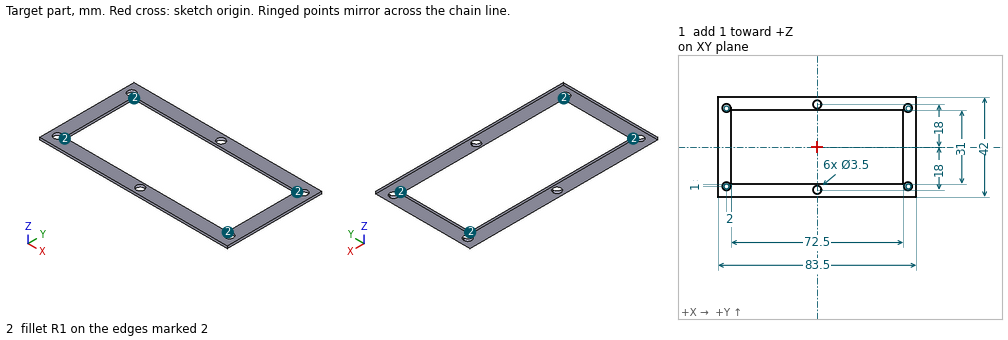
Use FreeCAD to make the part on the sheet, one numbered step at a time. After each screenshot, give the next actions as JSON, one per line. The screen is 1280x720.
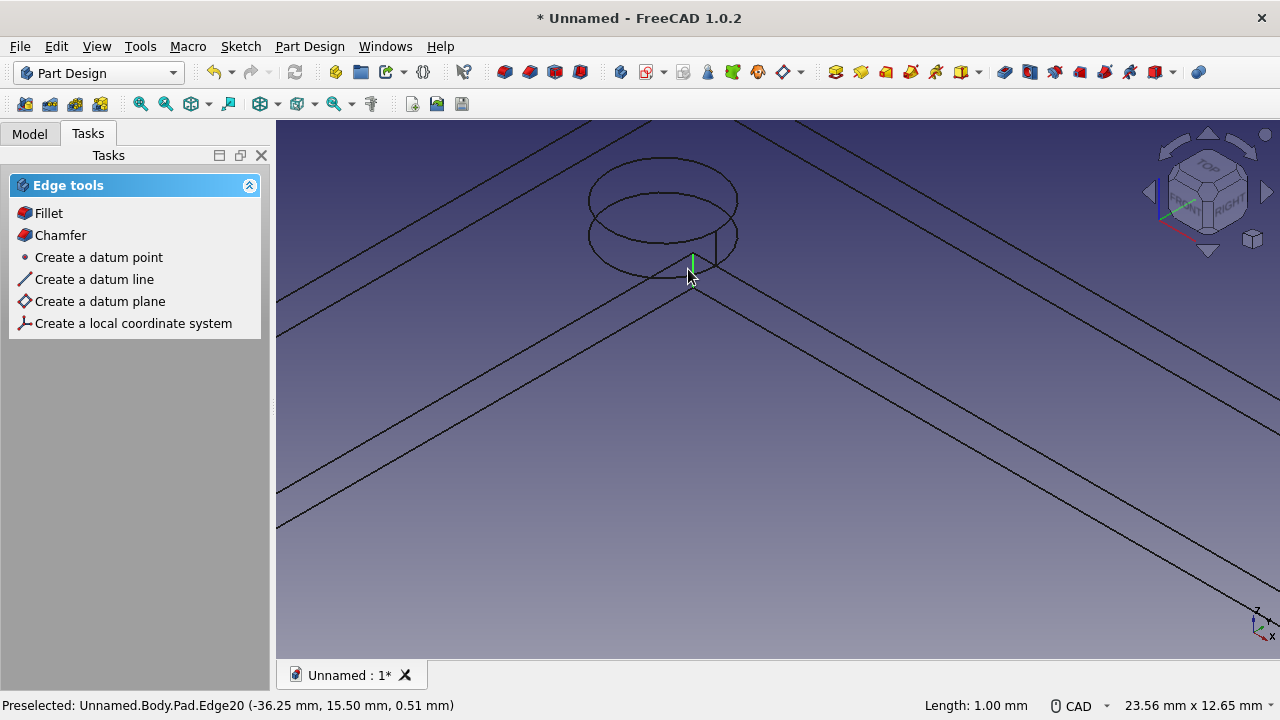
{"action": "key", "text": "v f"}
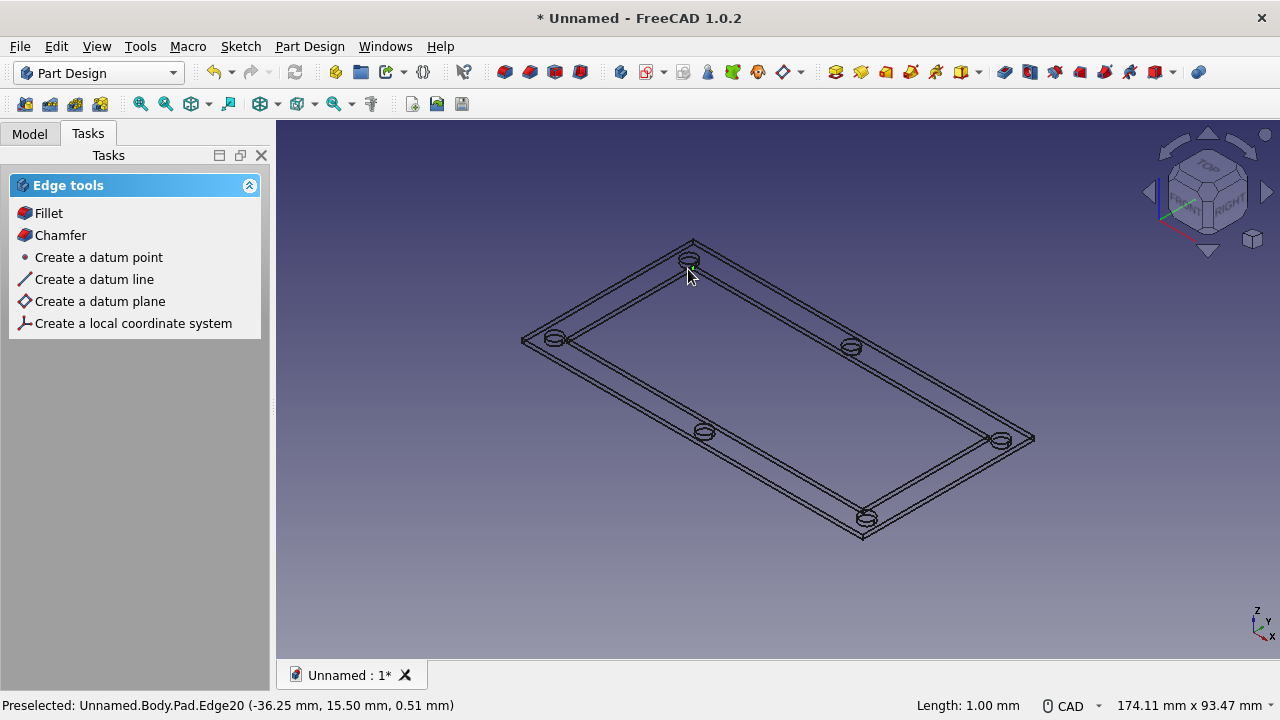
{"action": "key", "text": "2"}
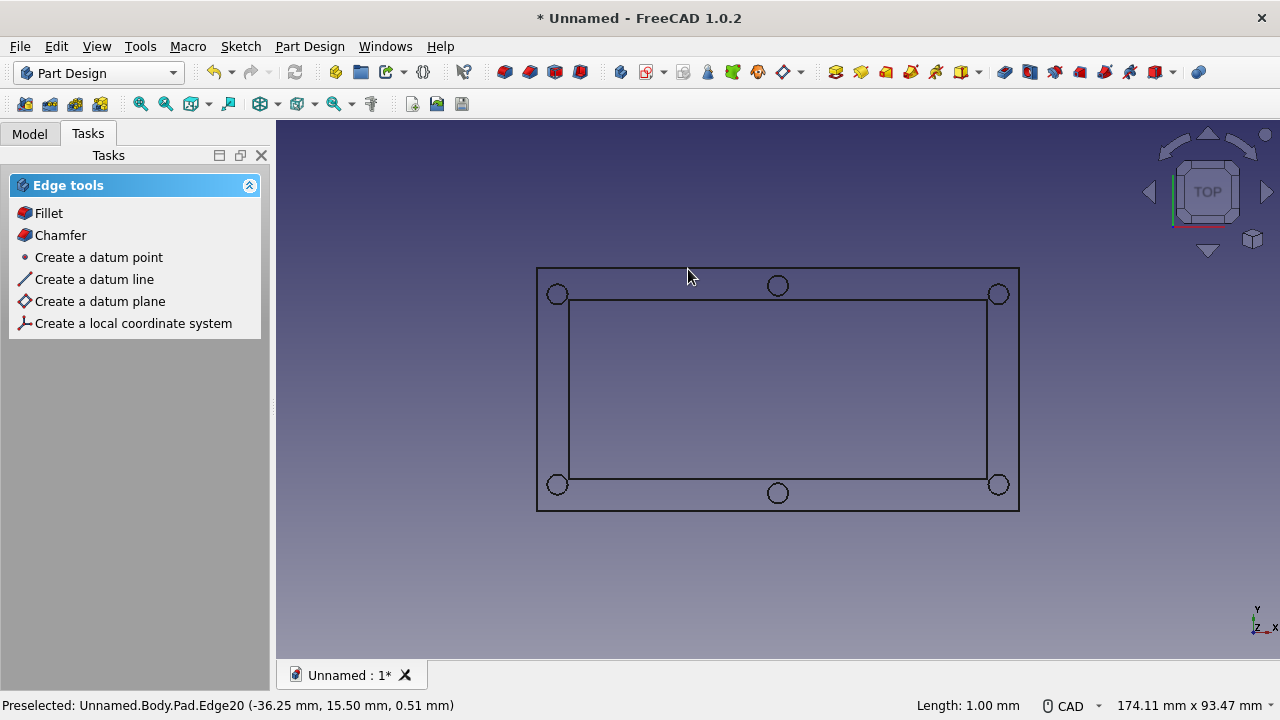
{"action": "scroll", "coordinate": [569, 478], "scroll_direction": "up", "scroll_amount": 10}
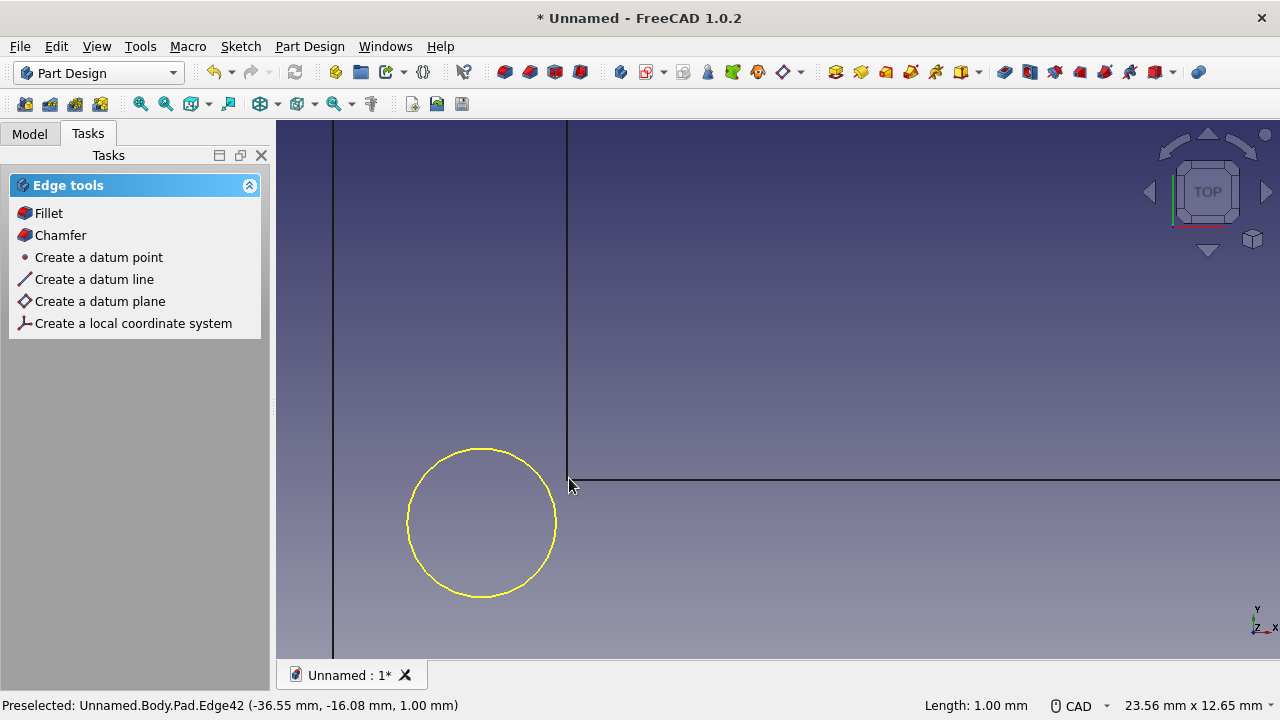
{"action": "left_click", "coordinate": [141, 104]}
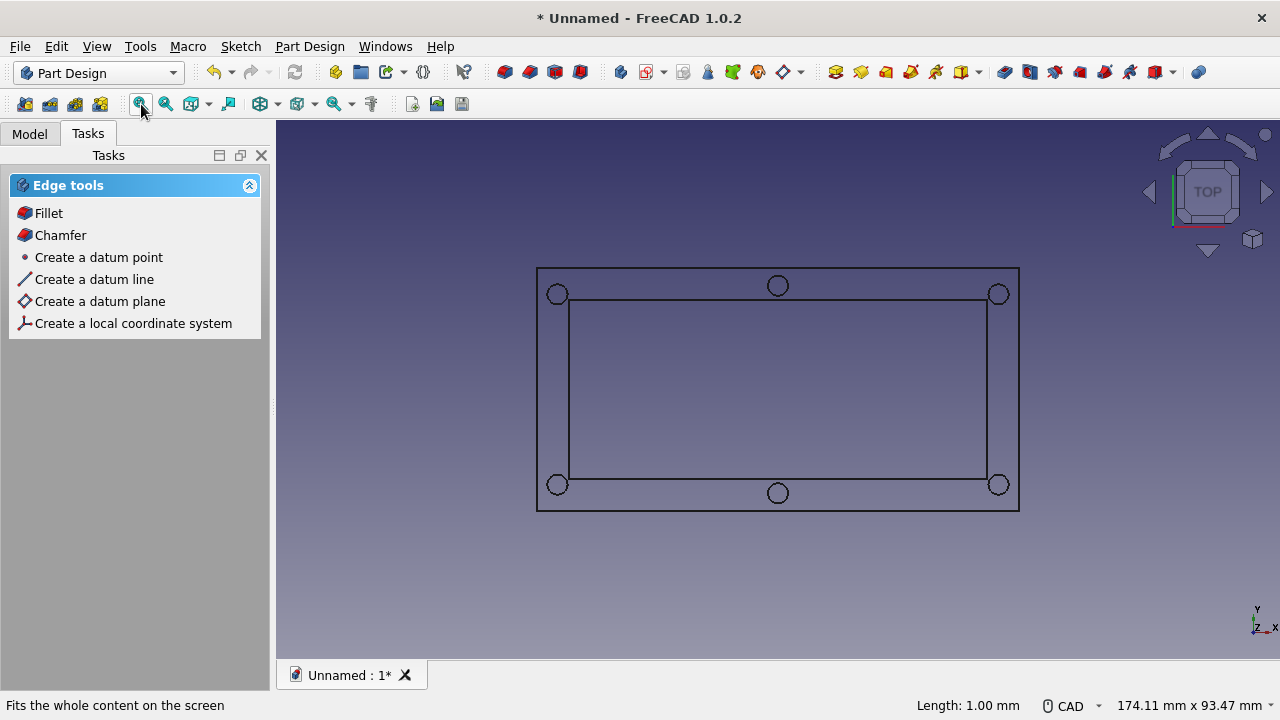
{"action": "key", "text": "1"}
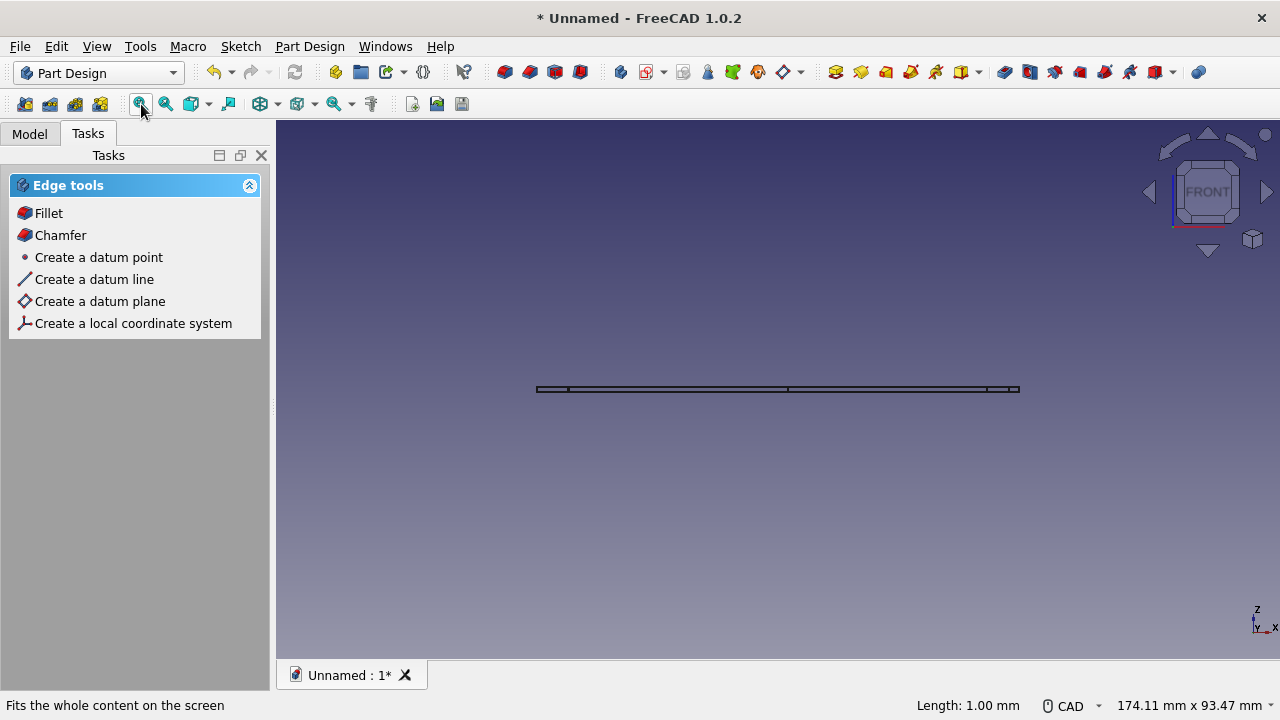
{"action": "scroll", "coordinate": [569, 389], "scroll_direction": "up", "scroll_amount": 10}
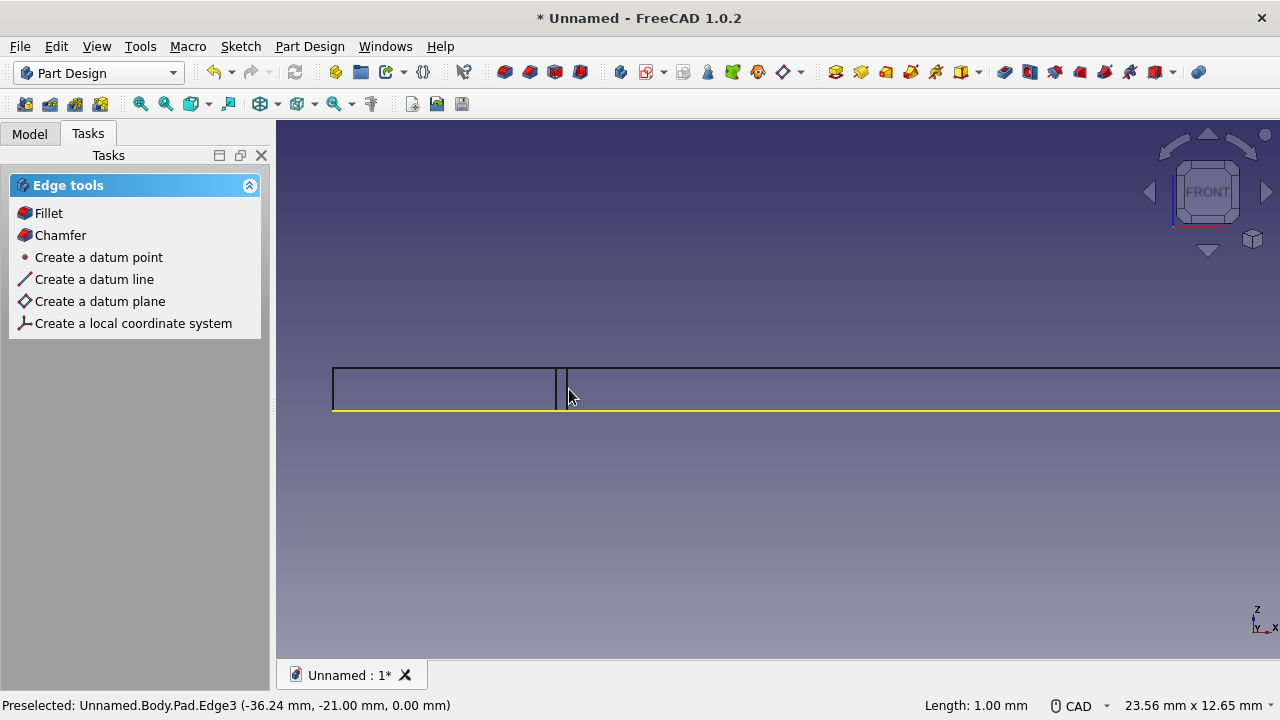
{"action": "left_click", "coordinate": [567, 389], "text": "ctrl"}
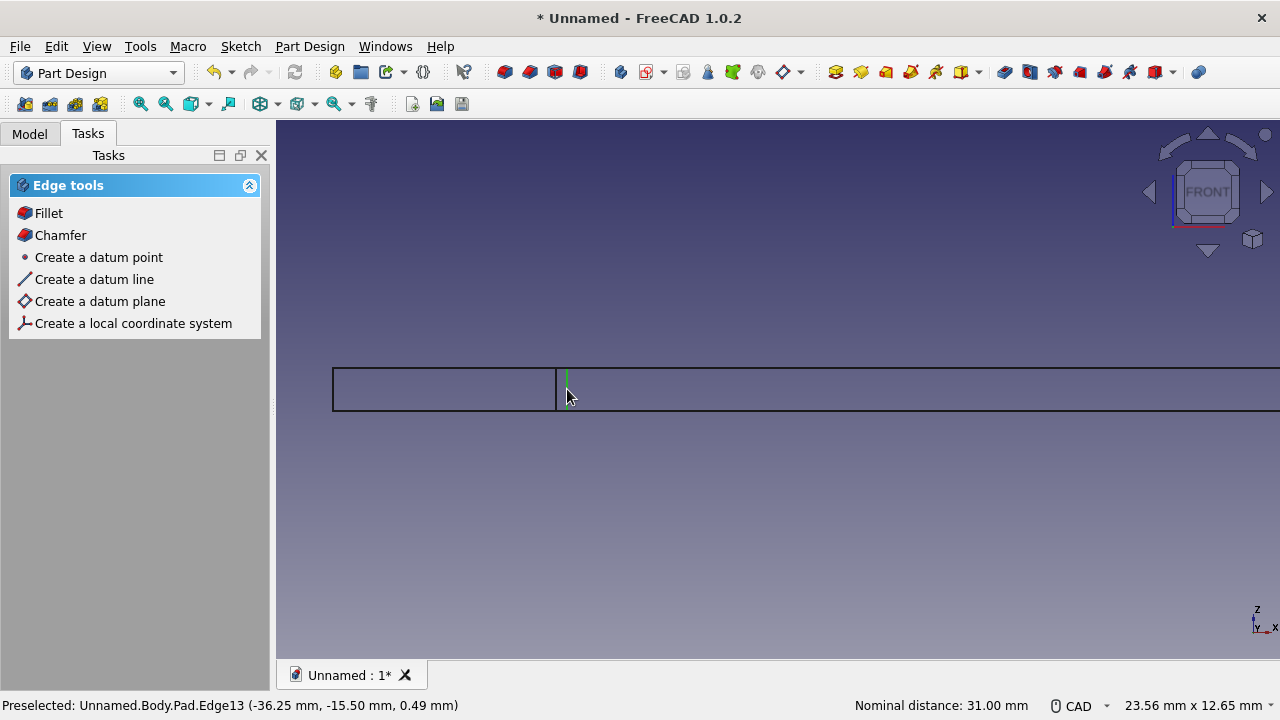
{"action": "key", "text": "v f"}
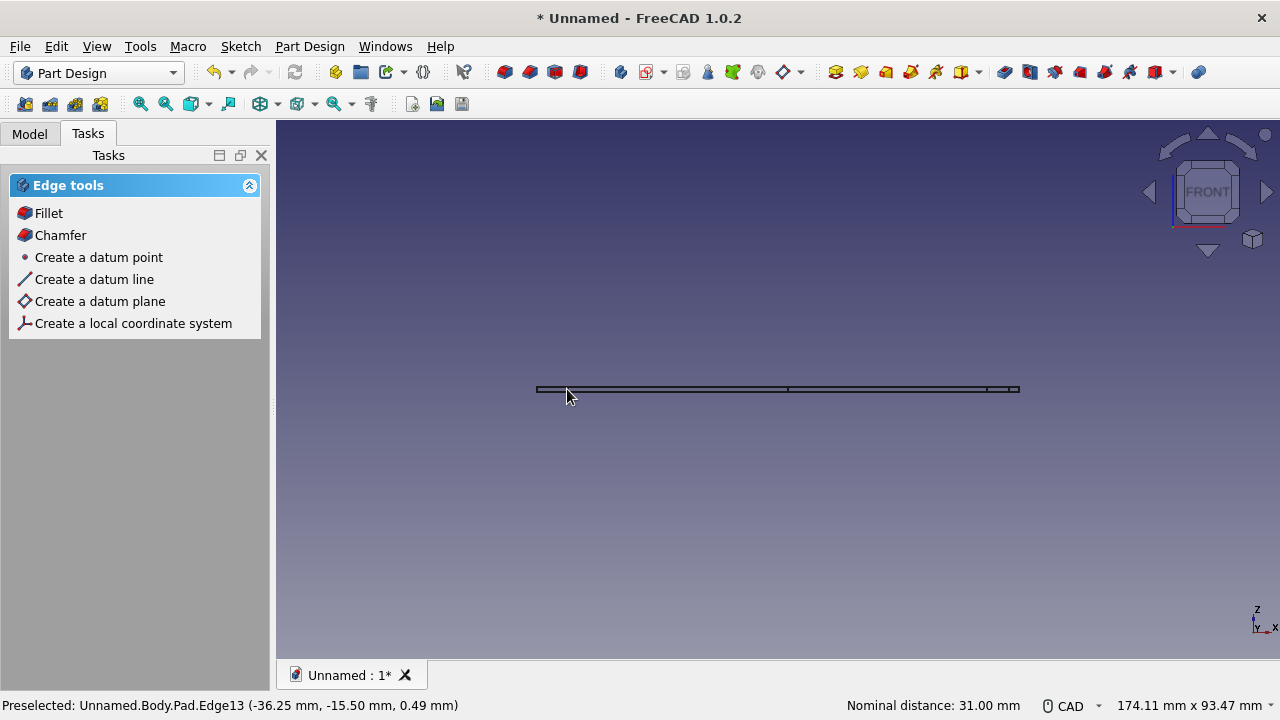
{"action": "key", "text": "3"}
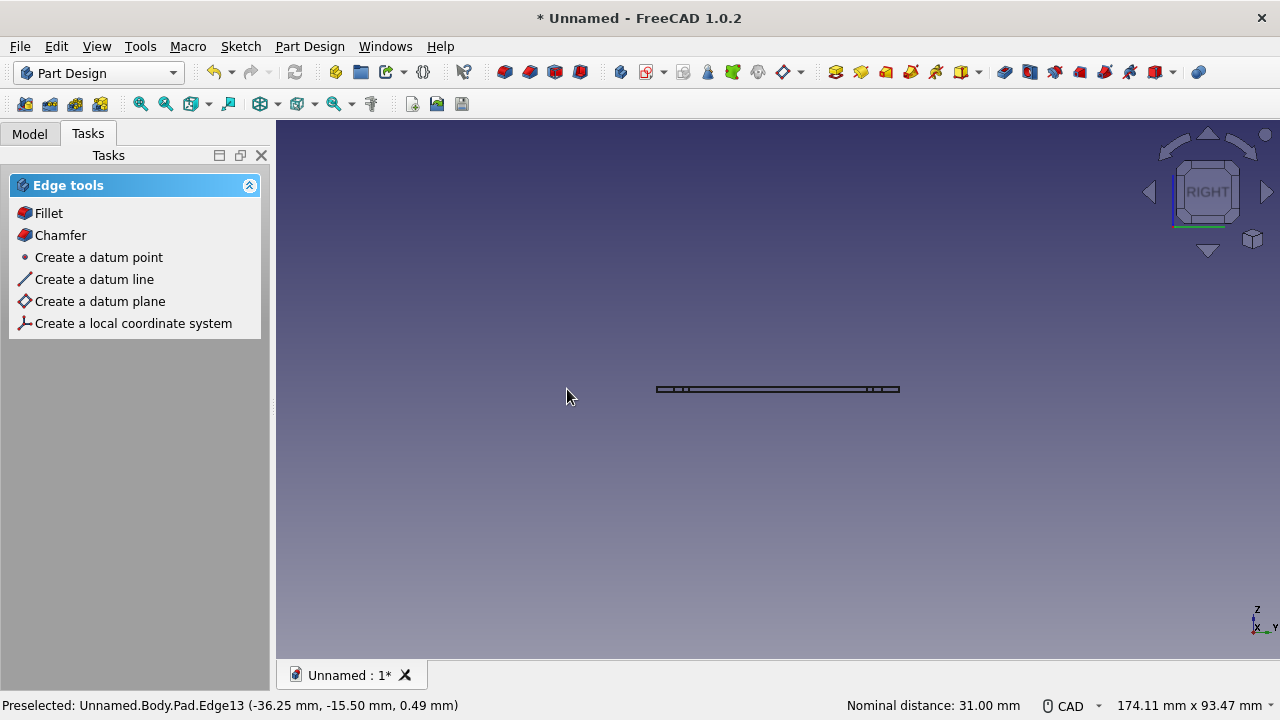
{"action": "key", "text": "v f"}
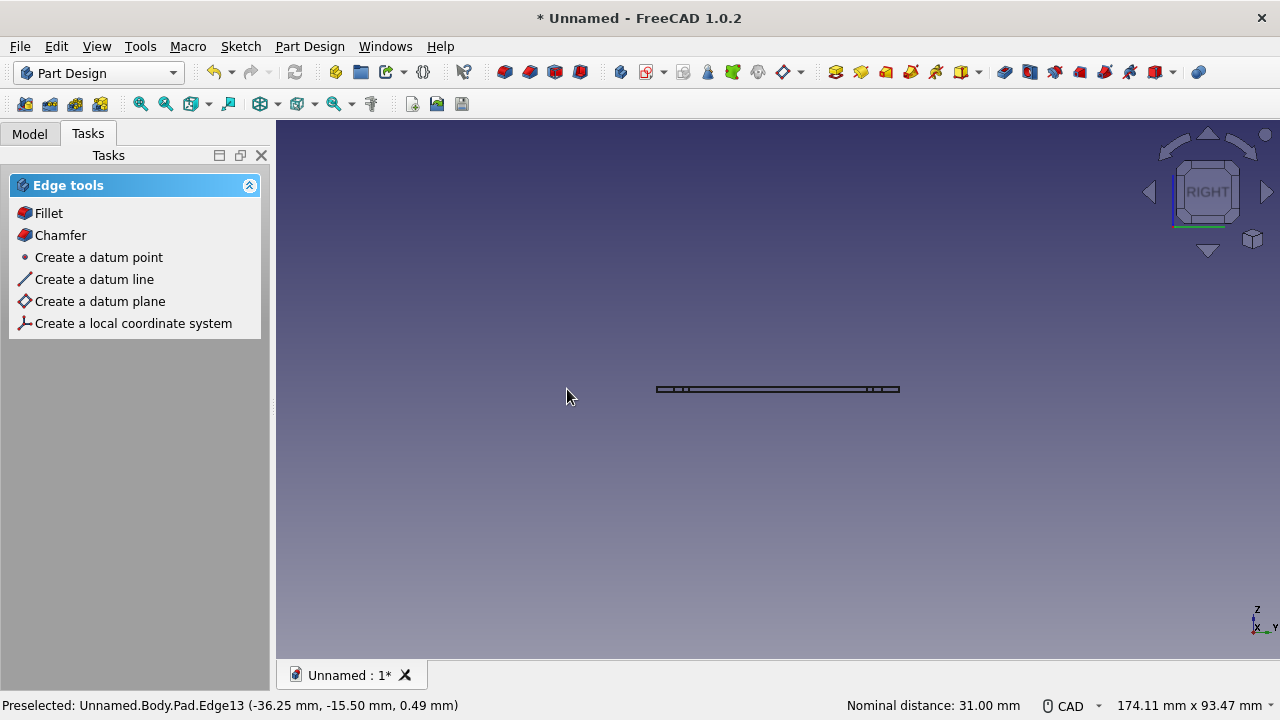
{"action": "scroll", "coordinate": [689, 388], "scroll_direction": "up", "scroll_amount": 10}